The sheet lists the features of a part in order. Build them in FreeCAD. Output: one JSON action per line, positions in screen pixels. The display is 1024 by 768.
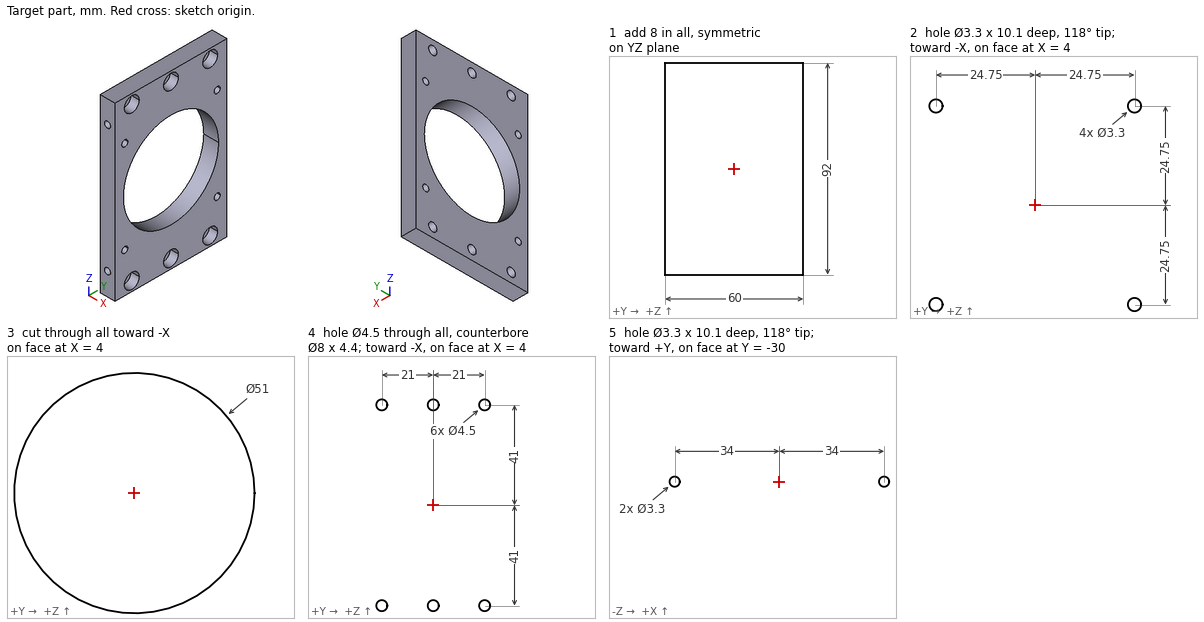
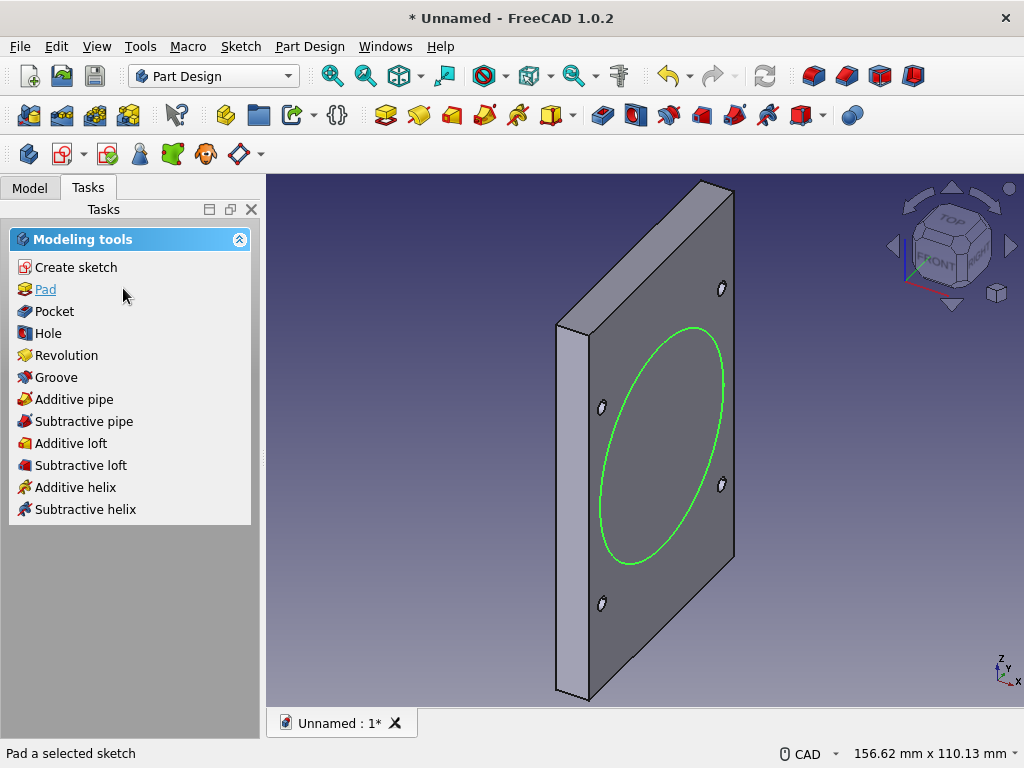
{"action": "left_click", "coordinate": [603, 116]}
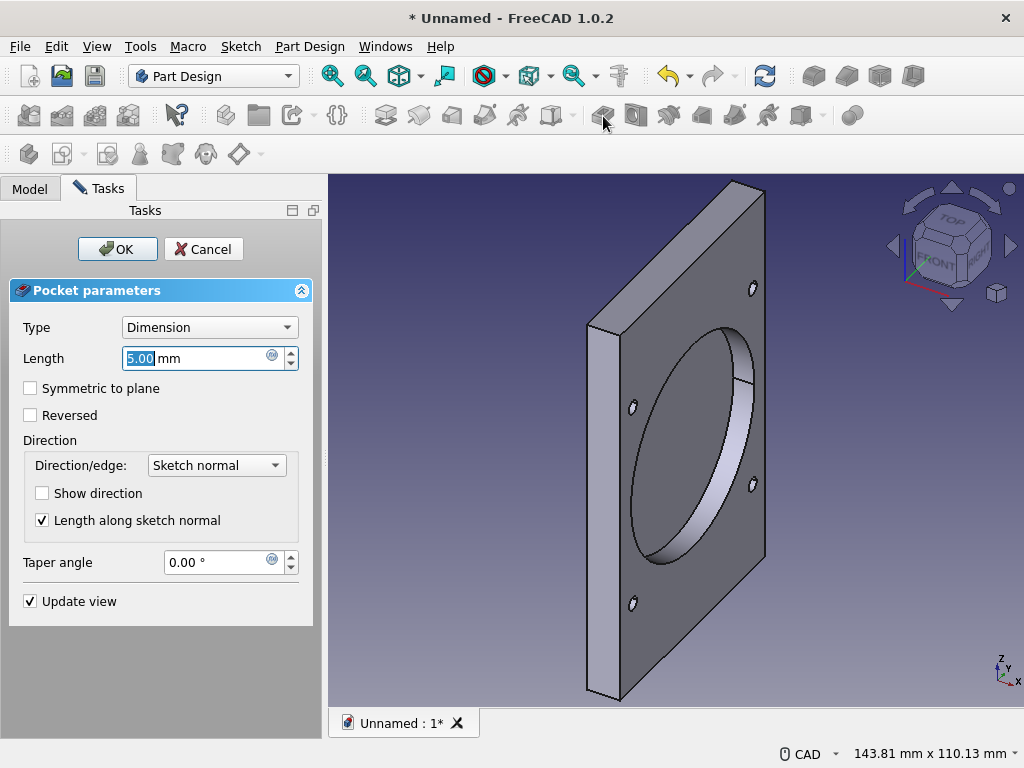
{"action": "left_click", "coordinate": [210, 328]}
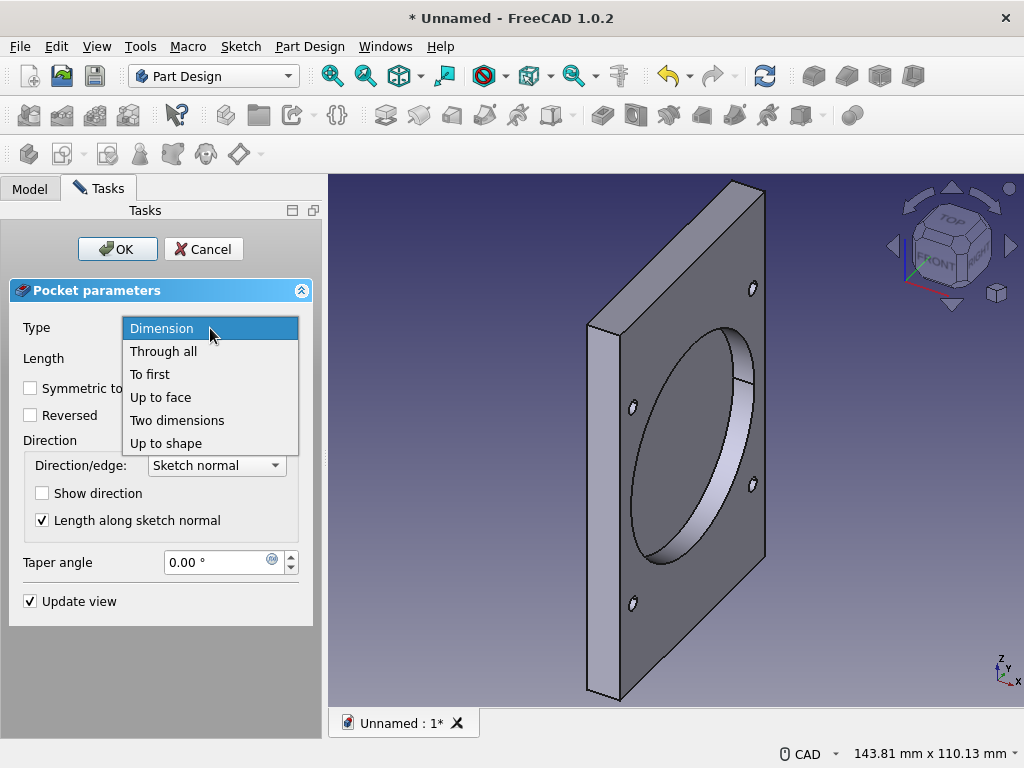
{"action": "left_click", "coordinate": [208, 352]}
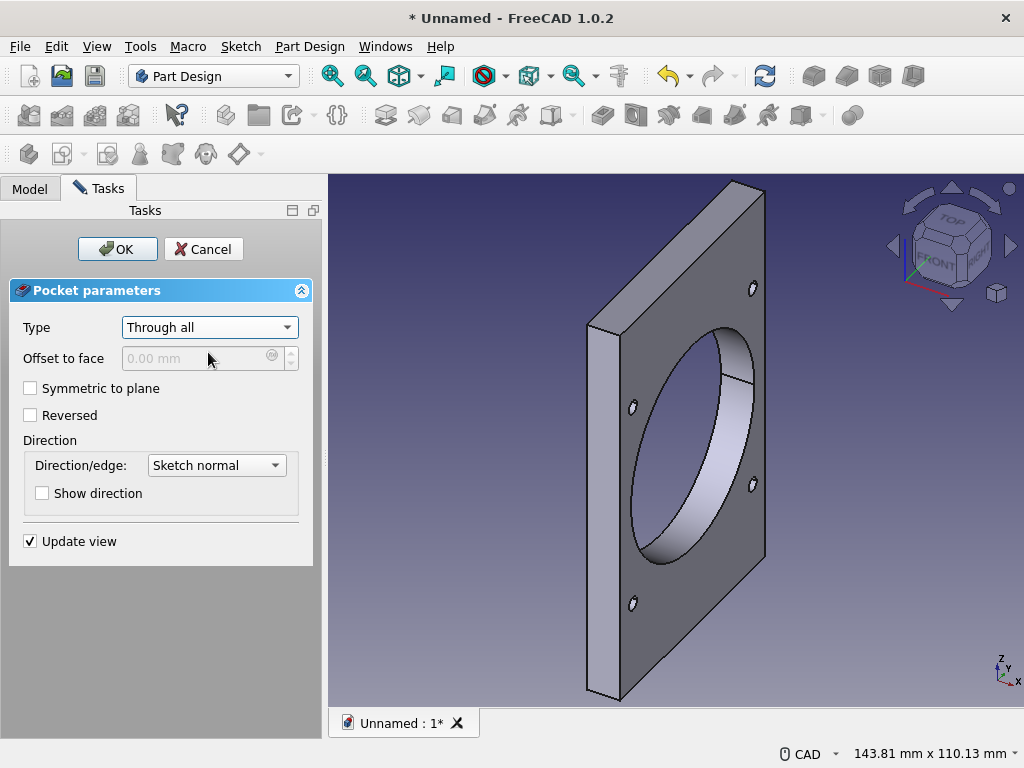
{"action": "left_click", "coordinate": [118, 249]}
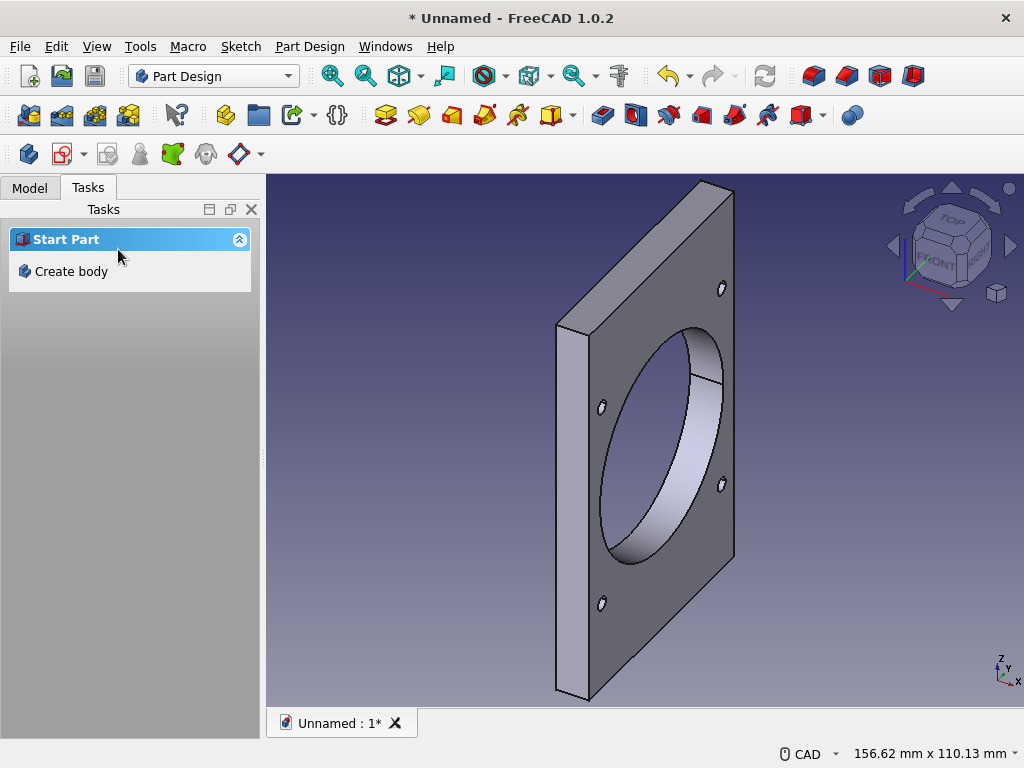
{"action": "left_click", "coordinate": [703, 560]}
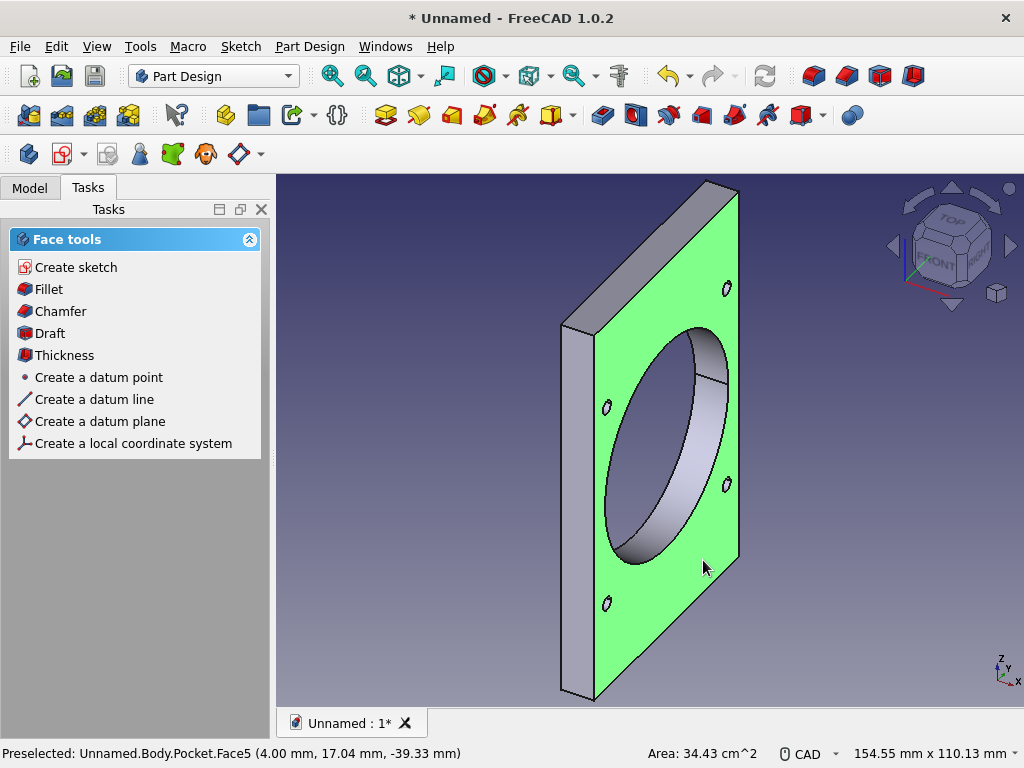
{"action": "left_click", "coordinate": [62, 154]}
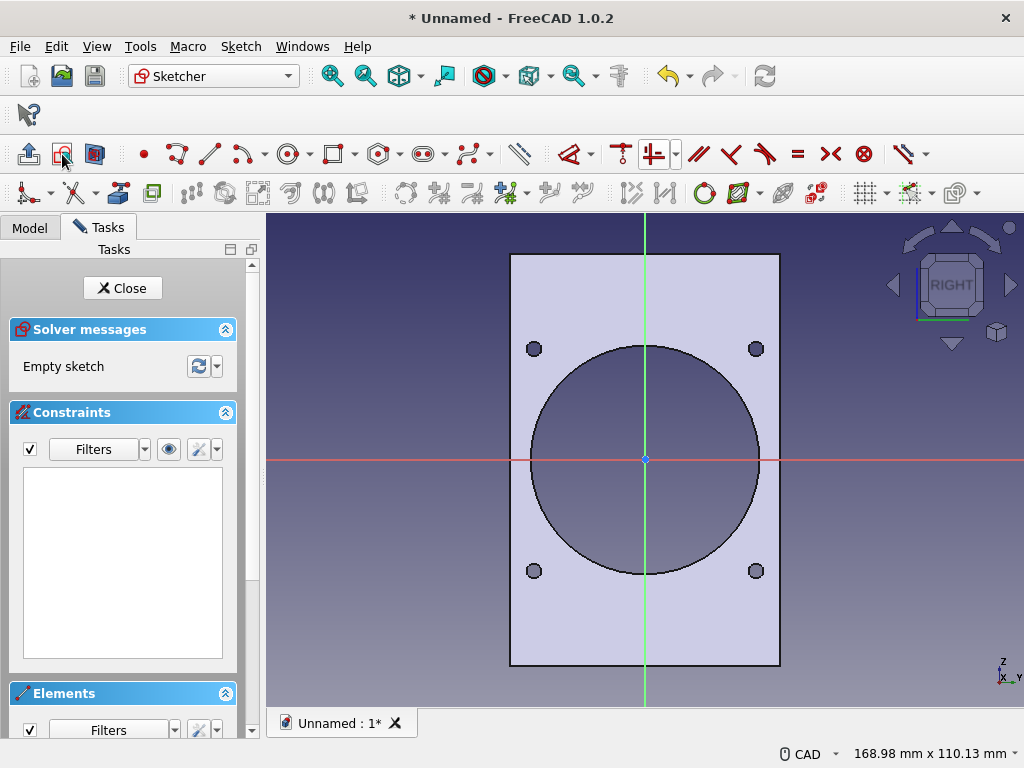
{"action": "scroll", "coordinate": [294, 460], "scroll_direction": "down", "scroll_amount": 1}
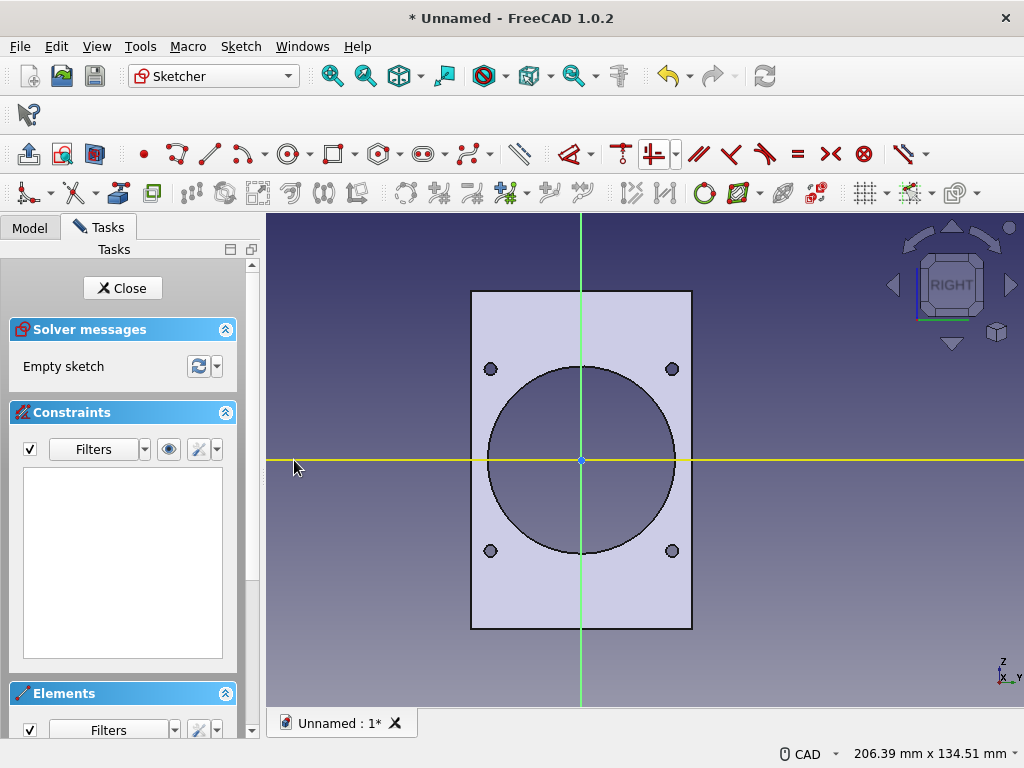
{"action": "left_click", "coordinate": [288, 154]}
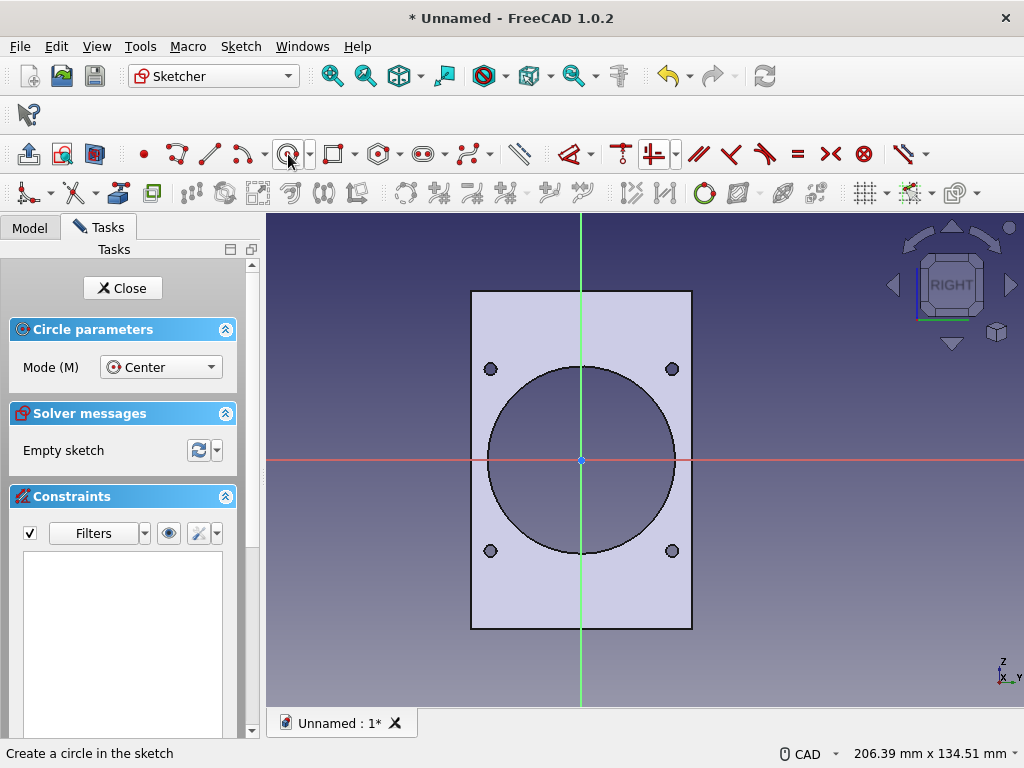
{"action": "scroll", "coordinate": [659, 310], "scroll_direction": "up", "scroll_amount": 6}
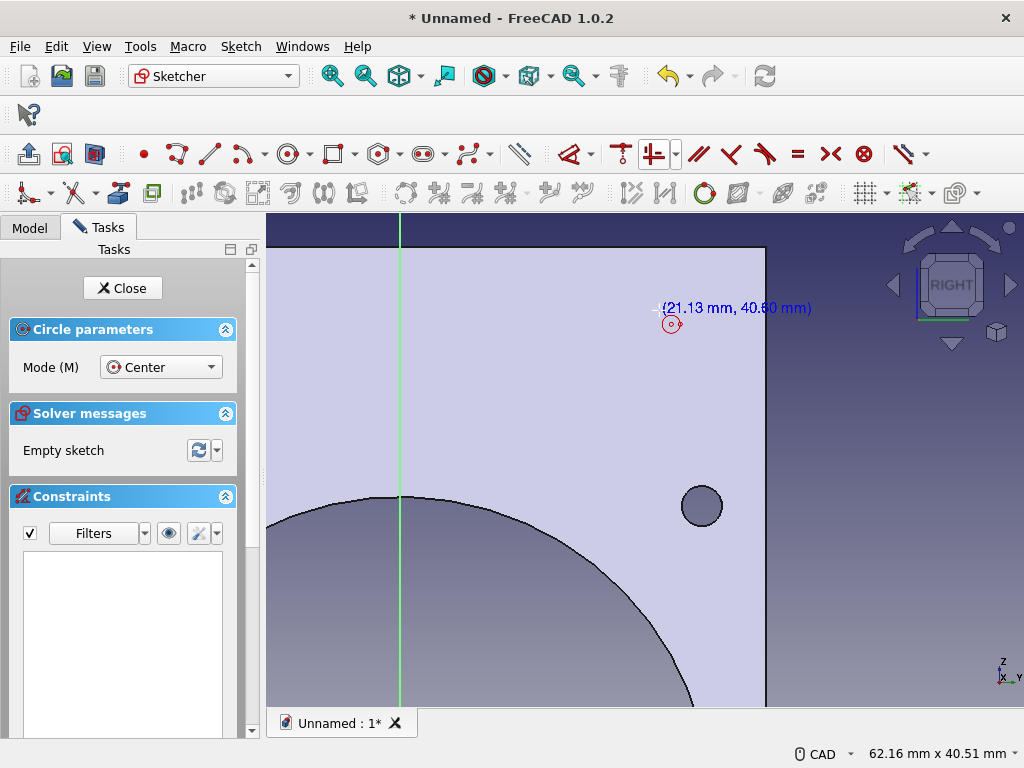
{"action": "left_click", "coordinate": [656, 308]}
{"action": "left_click", "coordinate": [676, 289]}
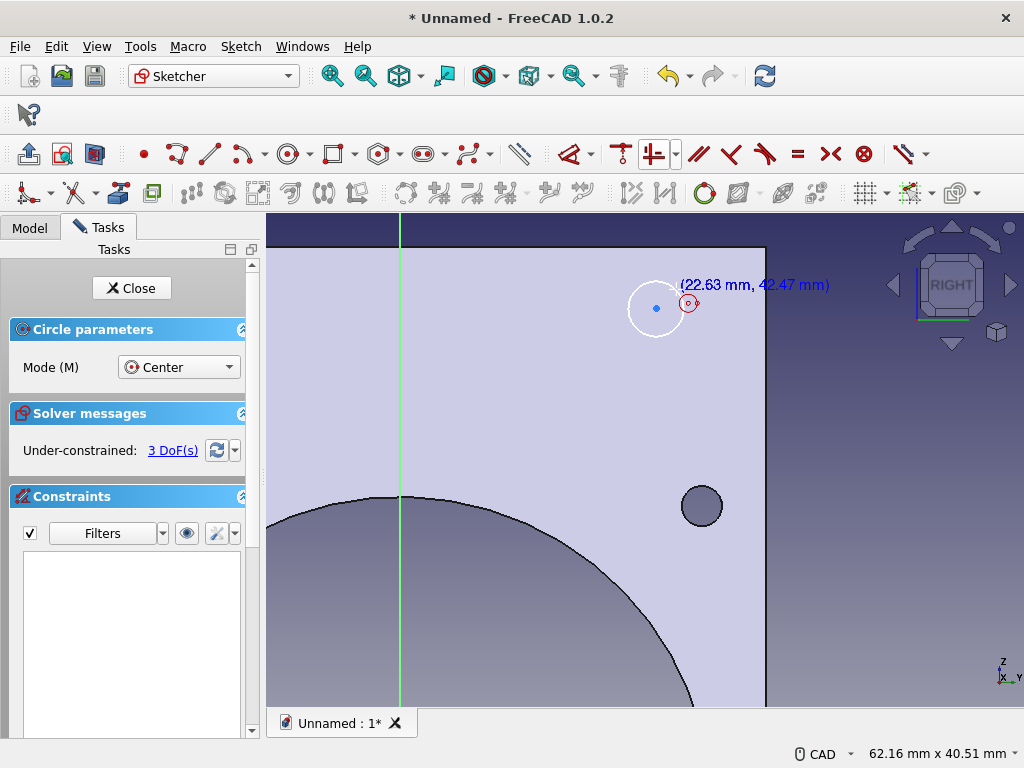
{"action": "left_click", "coordinate": [400, 308]}
{"action": "left_click", "coordinate": [419, 289]}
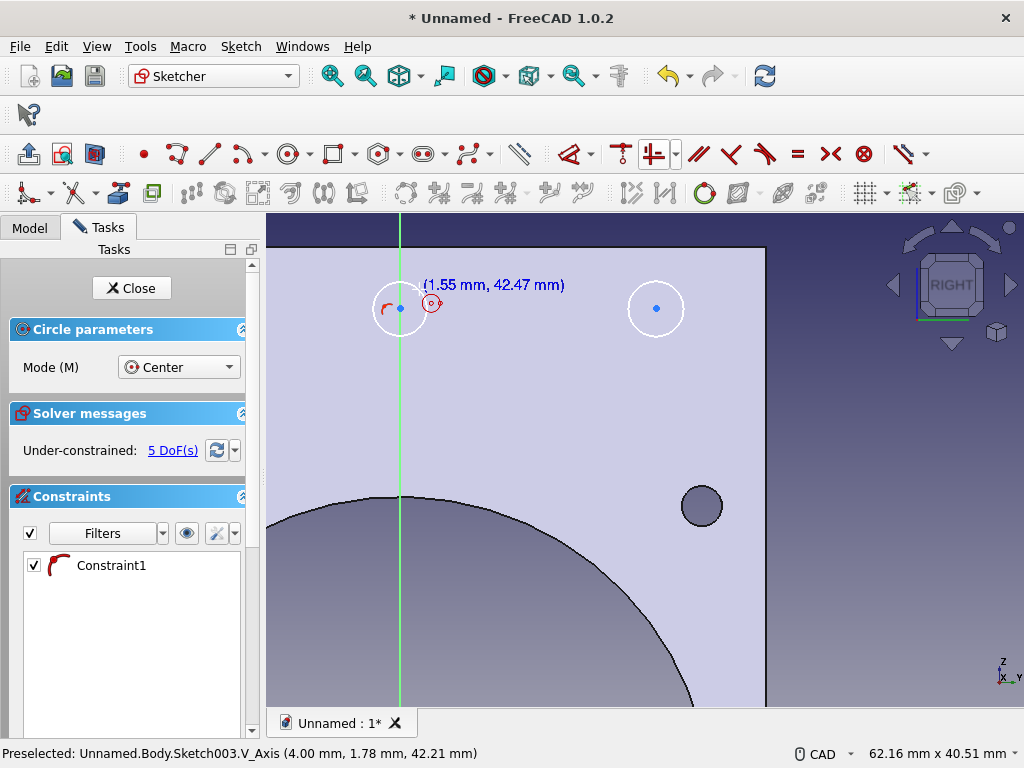
{"action": "scroll", "coordinate": [653, 310], "scroll_direction": "down", "scroll_amount": 6}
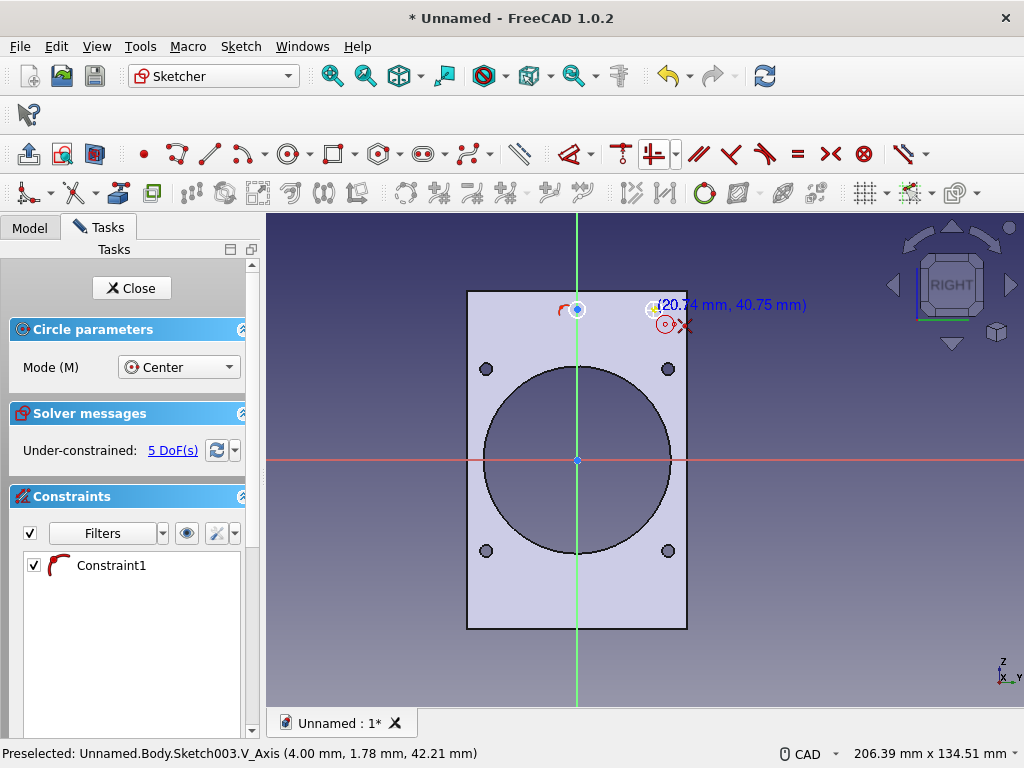
{"action": "scroll", "coordinate": [500, 310], "scroll_direction": "up", "scroll_amount": 6}